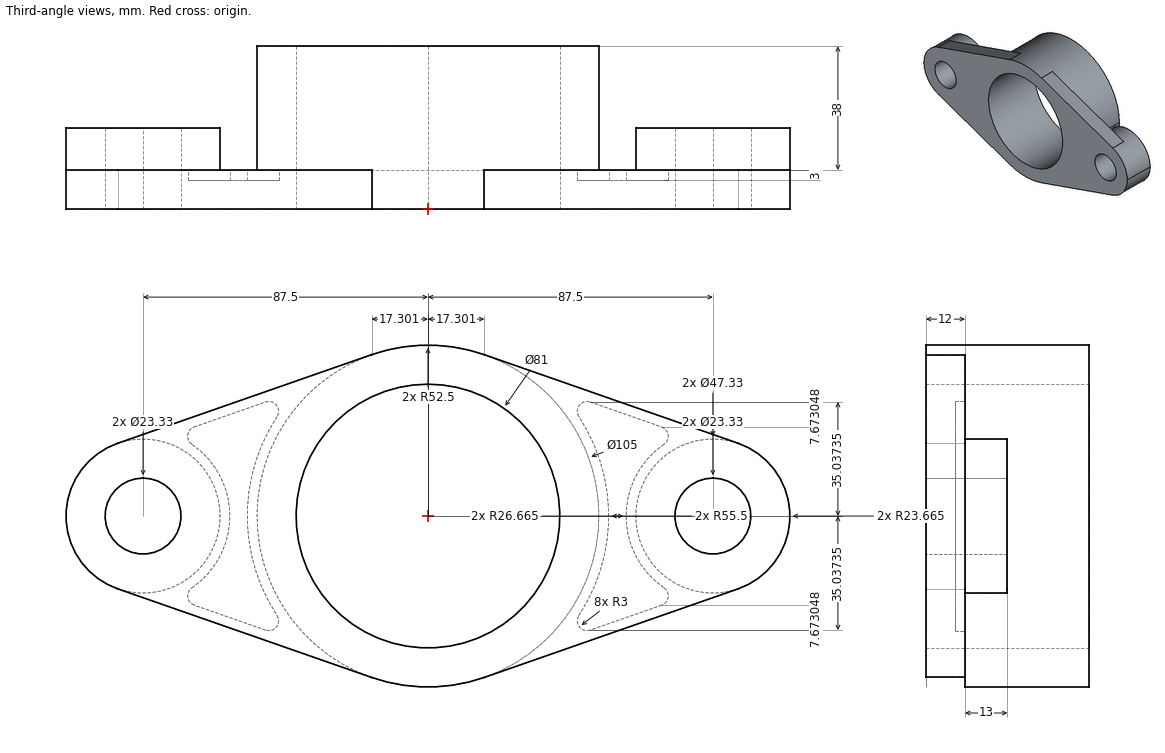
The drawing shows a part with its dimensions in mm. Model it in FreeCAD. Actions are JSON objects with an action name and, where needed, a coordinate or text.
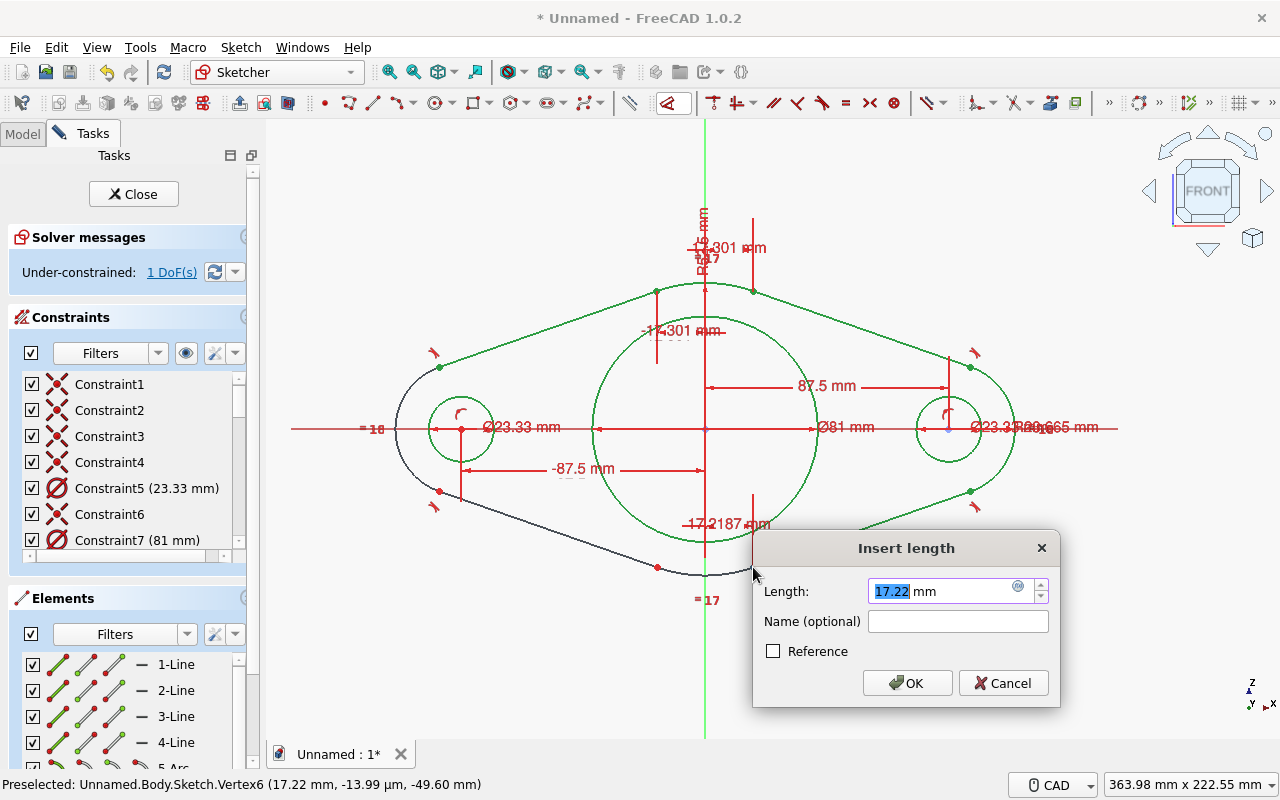
{"action": "type", "text": "17.301"}
{"action": "key", "text": "Return"}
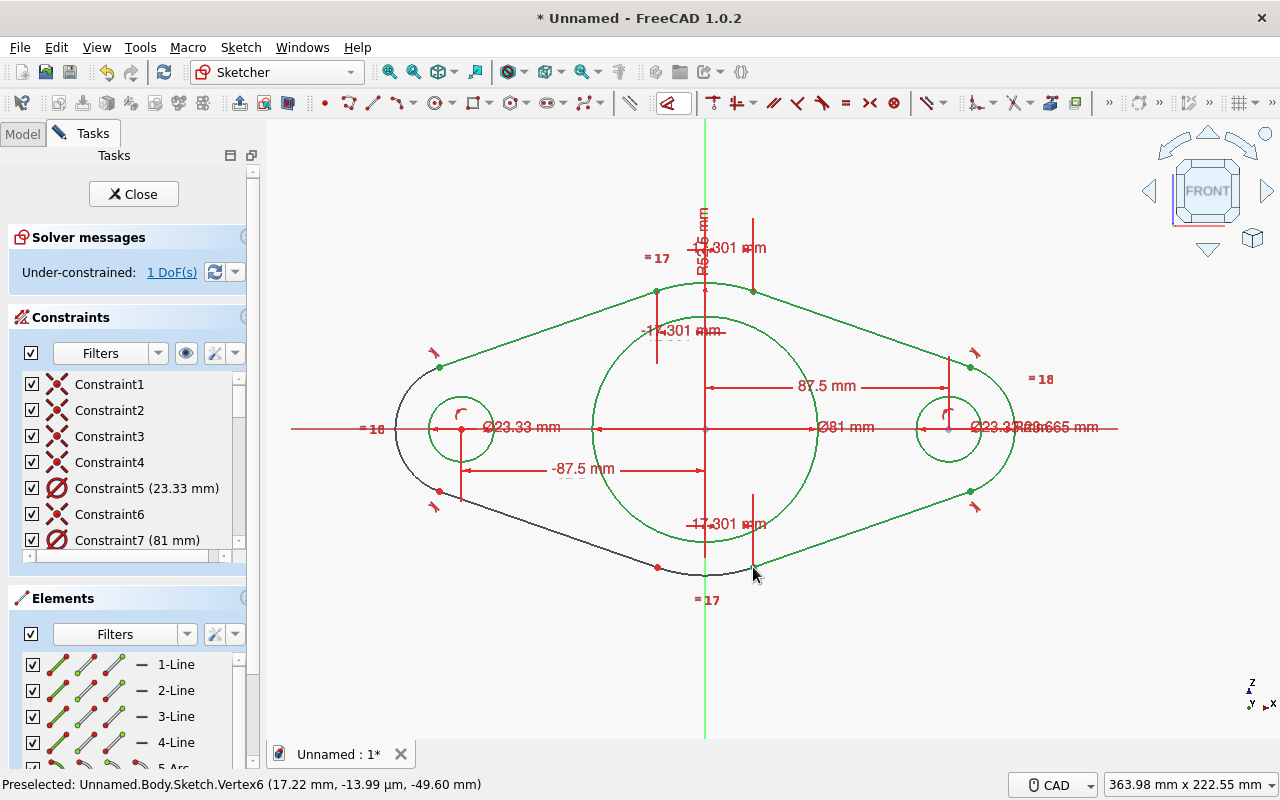
{"action": "left_click", "coordinate": [657, 567]}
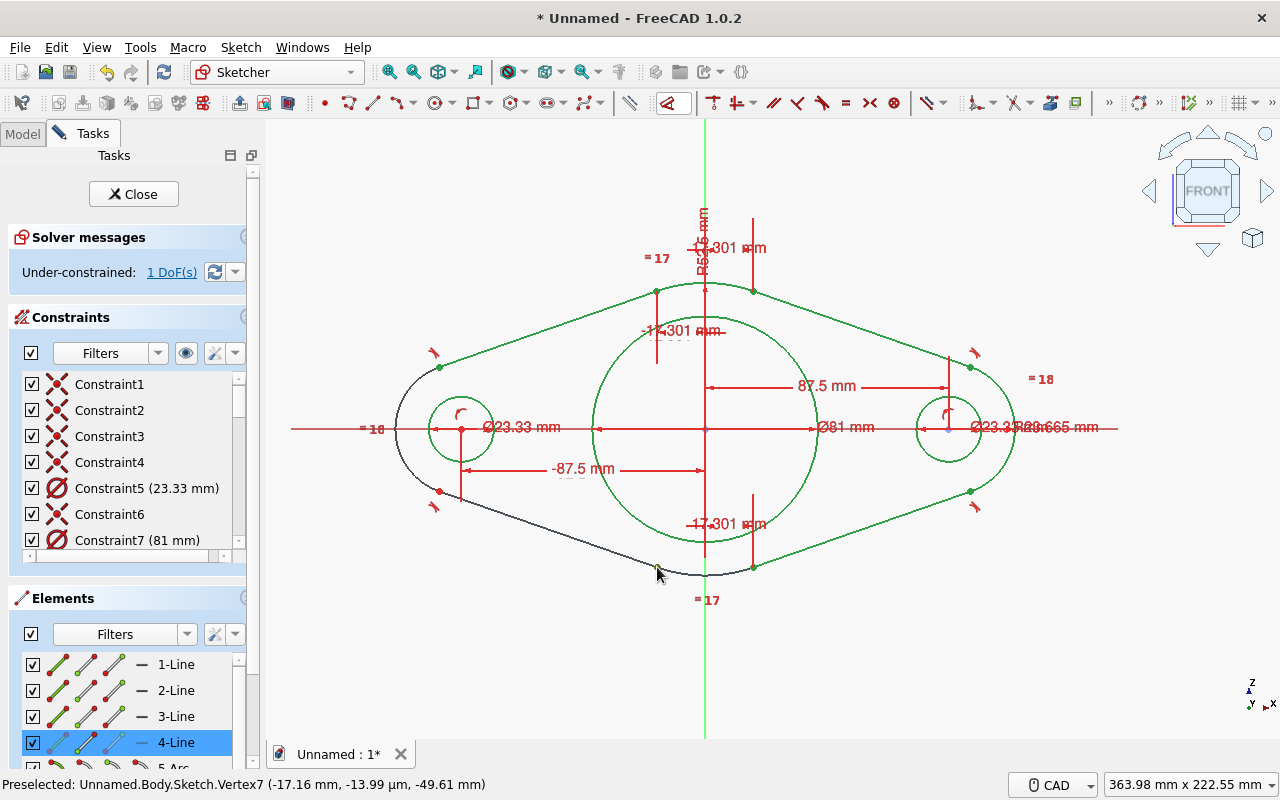
{"action": "key", "text": "l"}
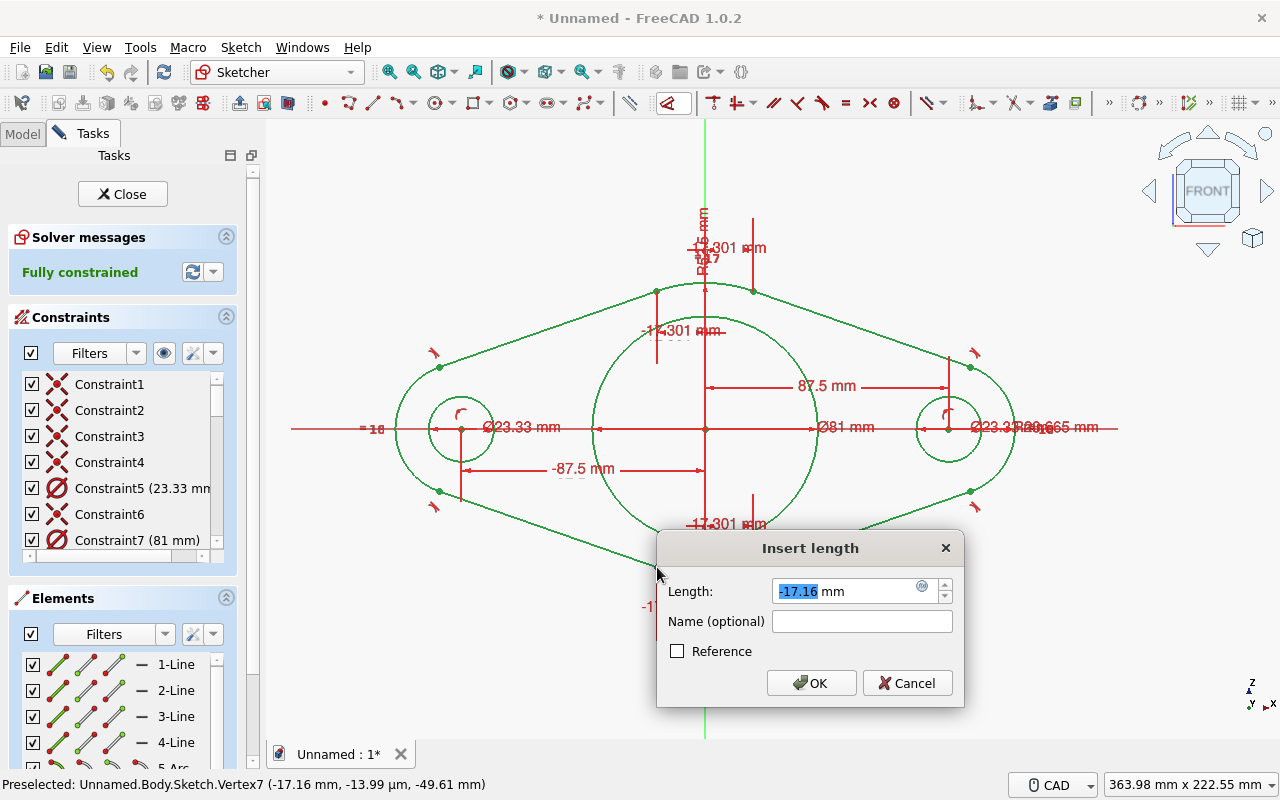
{"action": "type", "text": "-17.301"}
{"action": "key", "text": "Return"}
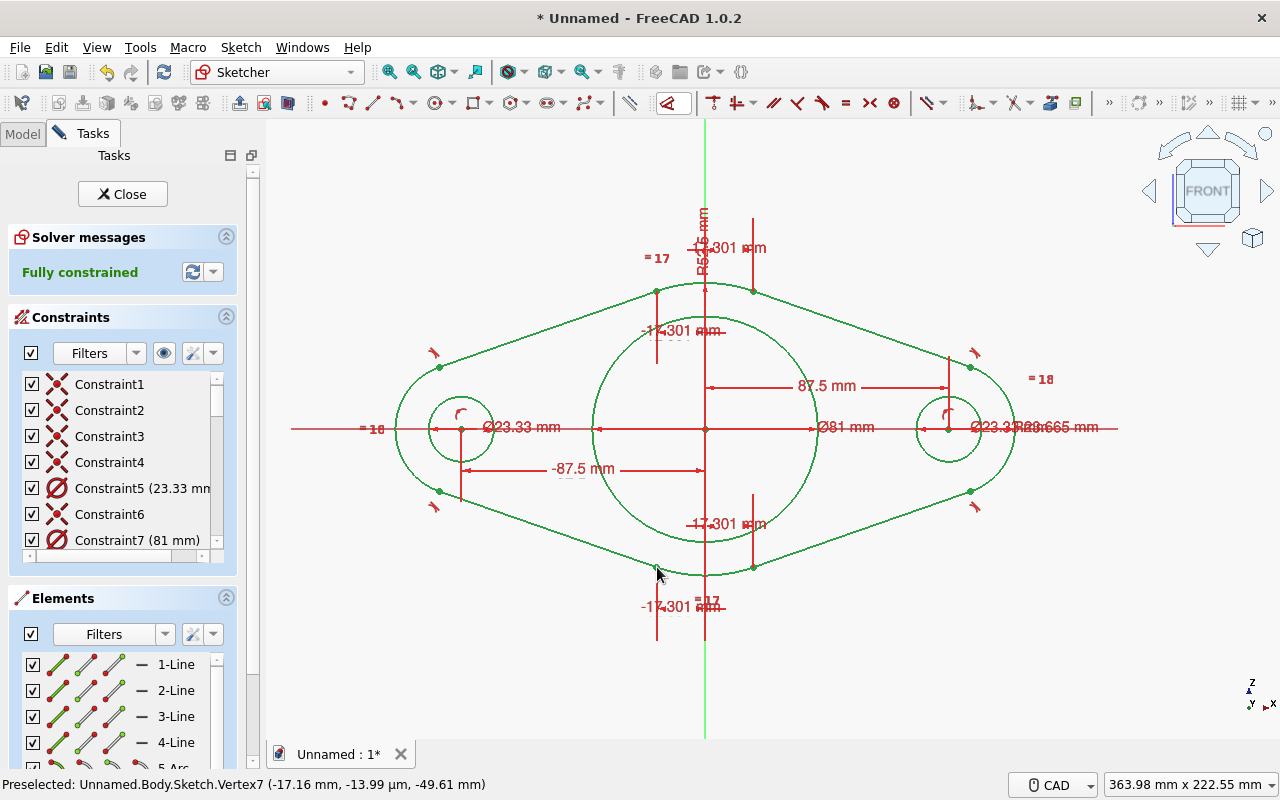
{"action": "left_click", "coordinate": [123, 194]}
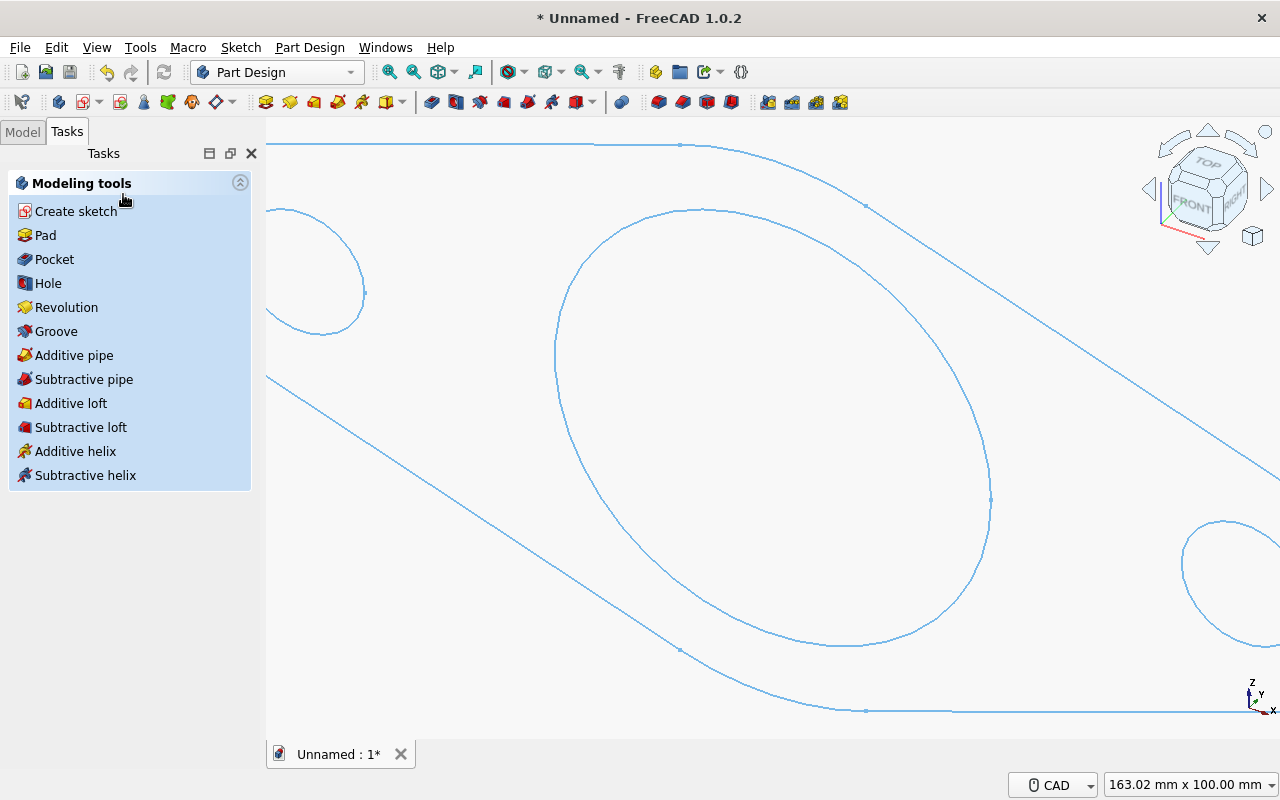
{"action": "left_click", "coordinate": [266, 102]}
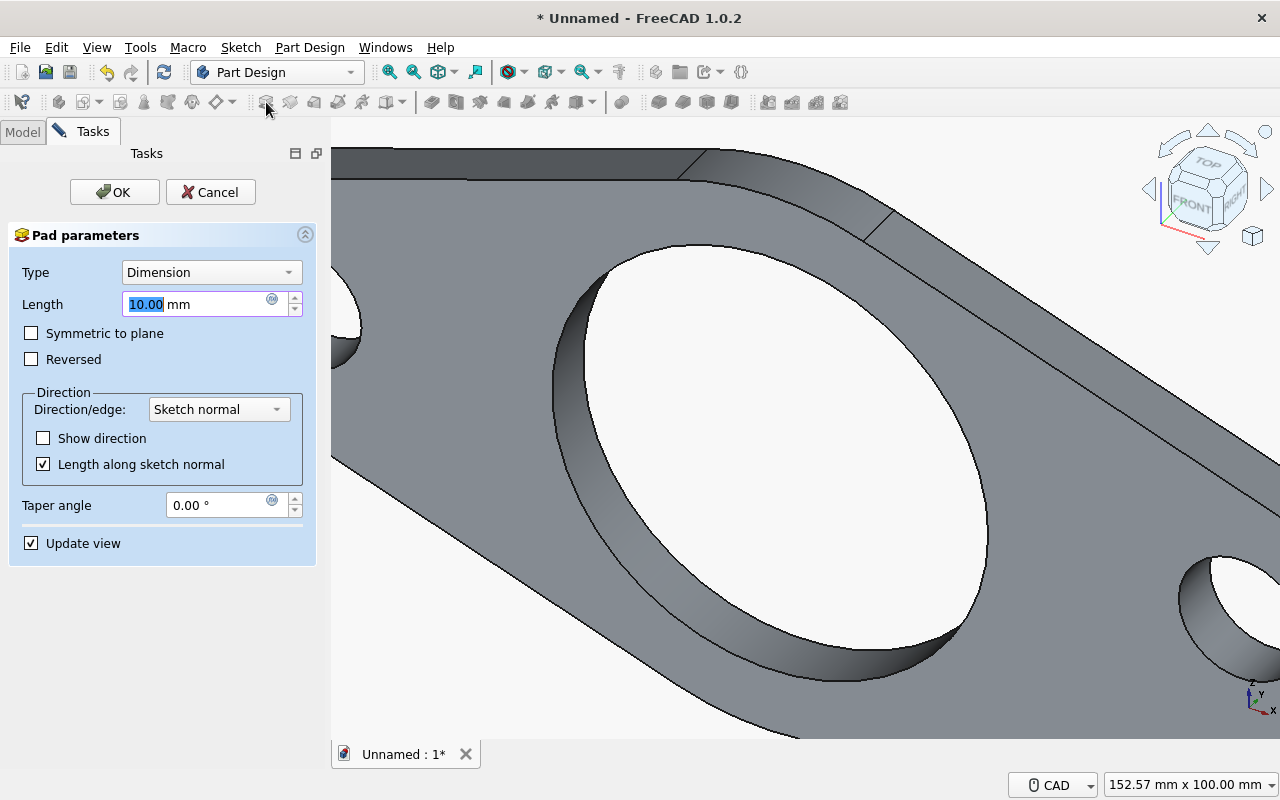
{"action": "type", "text": "12"}
{"action": "key", "text": "Tab"}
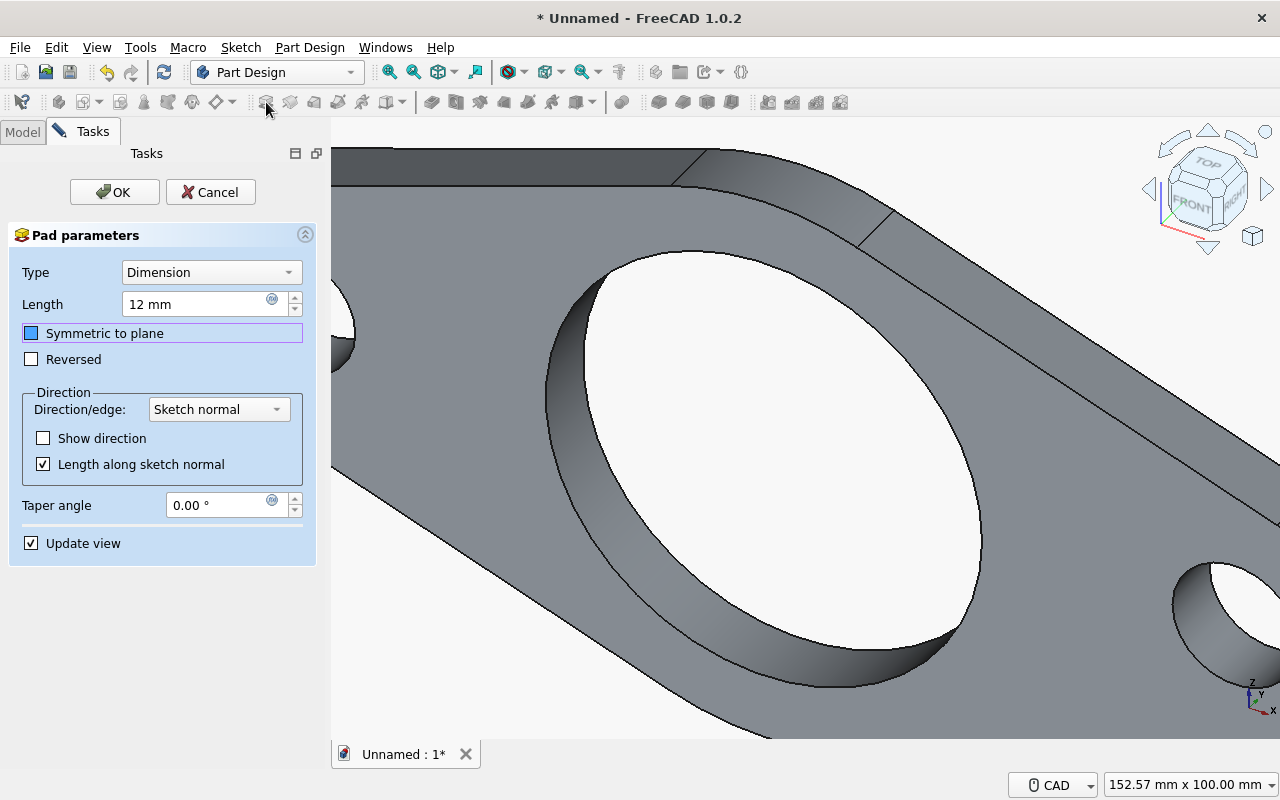
{"action": "left_click", "coordinate": [30, 359]}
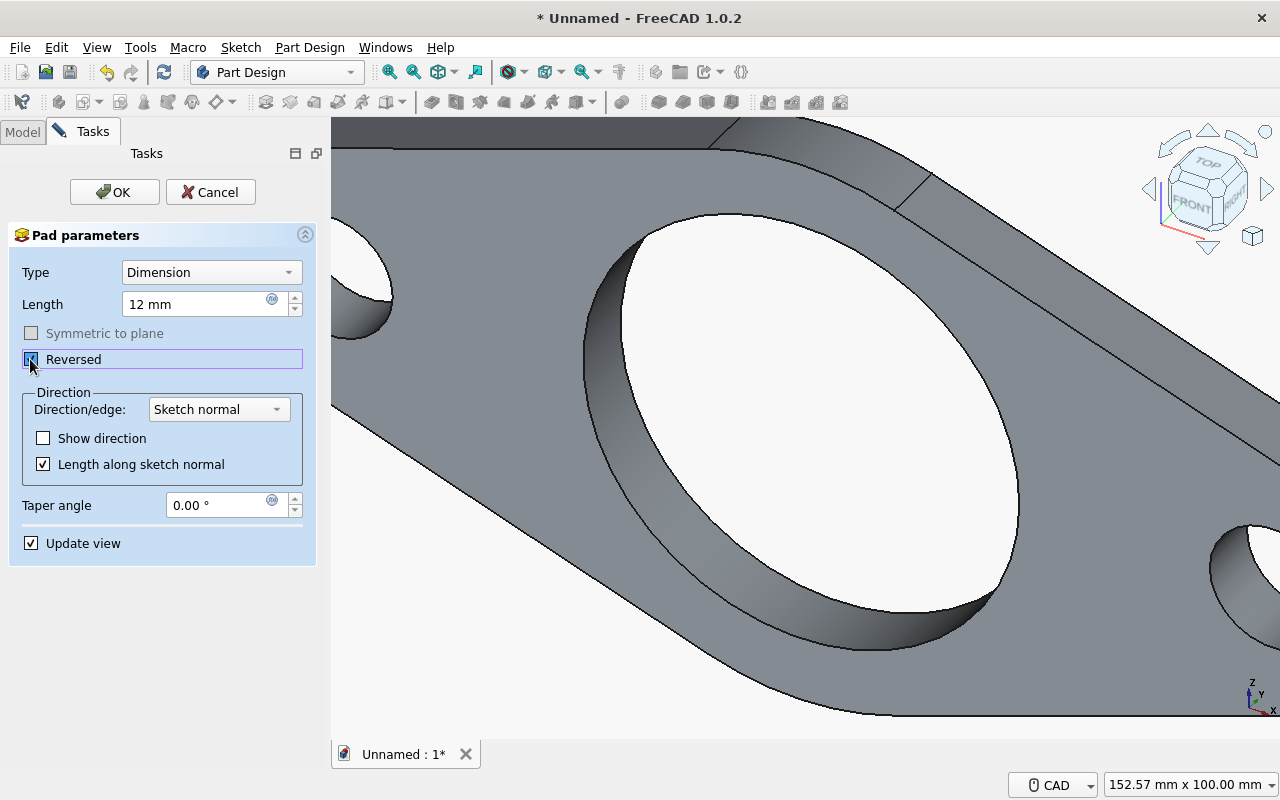
{"action": "left_click", "coordinate": [115, 192]}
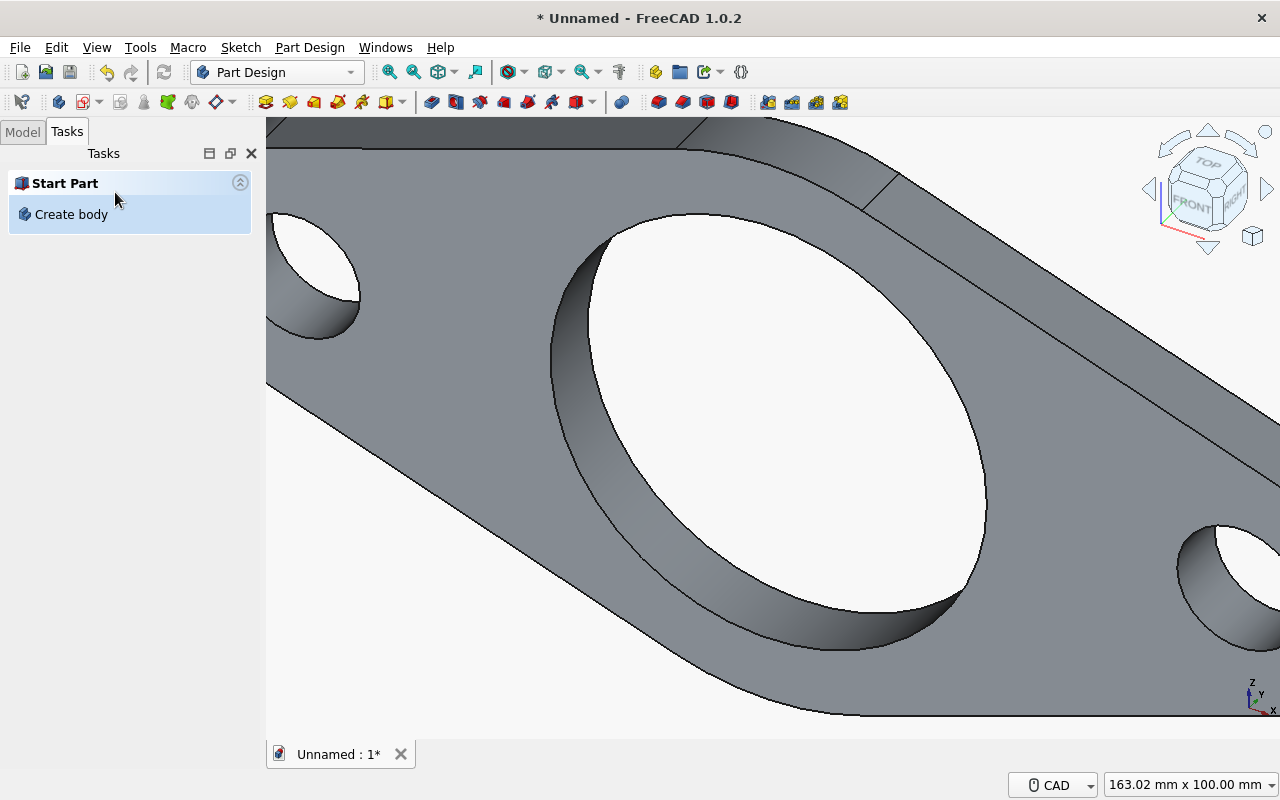
{"action": "left_click", "coordinate": [390, 72]}